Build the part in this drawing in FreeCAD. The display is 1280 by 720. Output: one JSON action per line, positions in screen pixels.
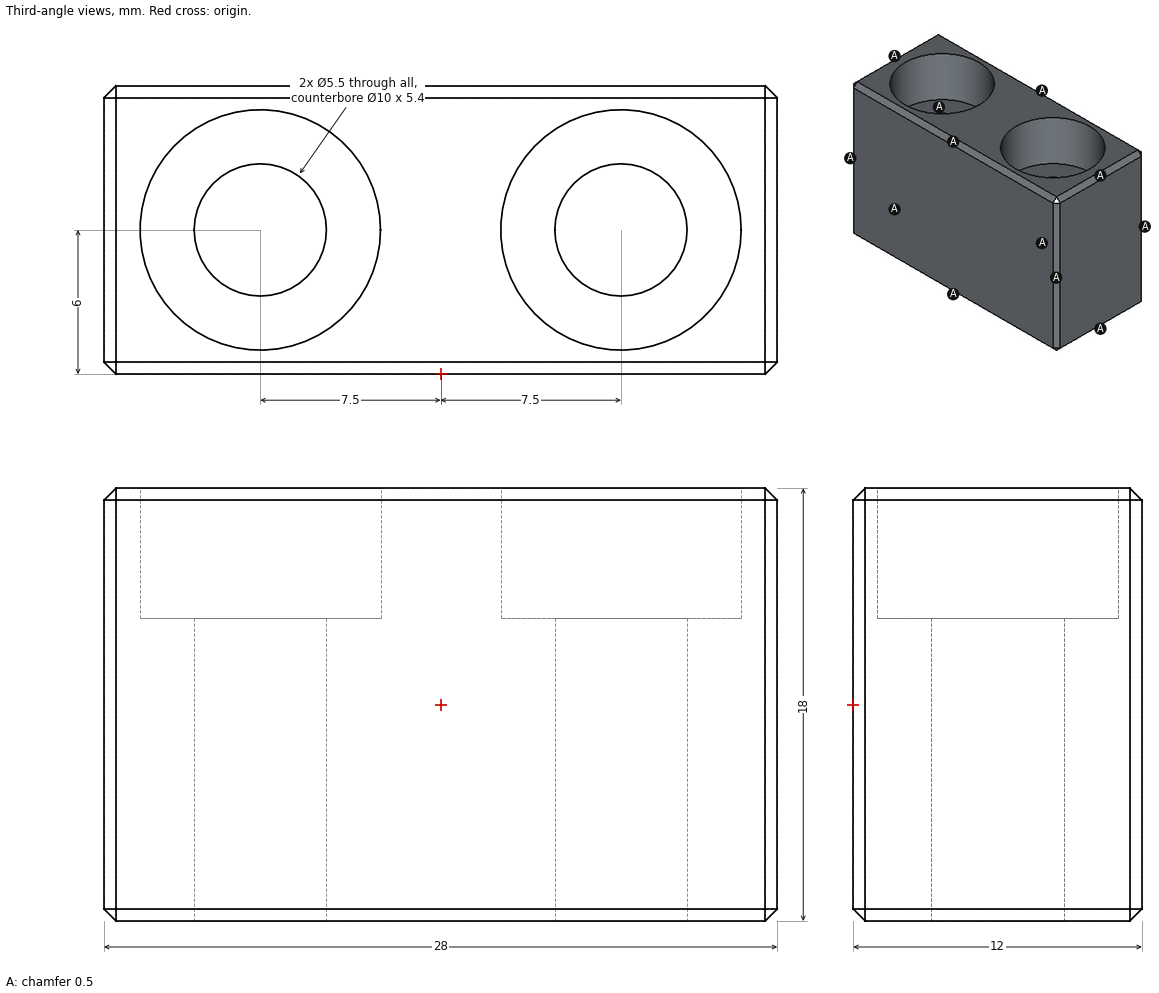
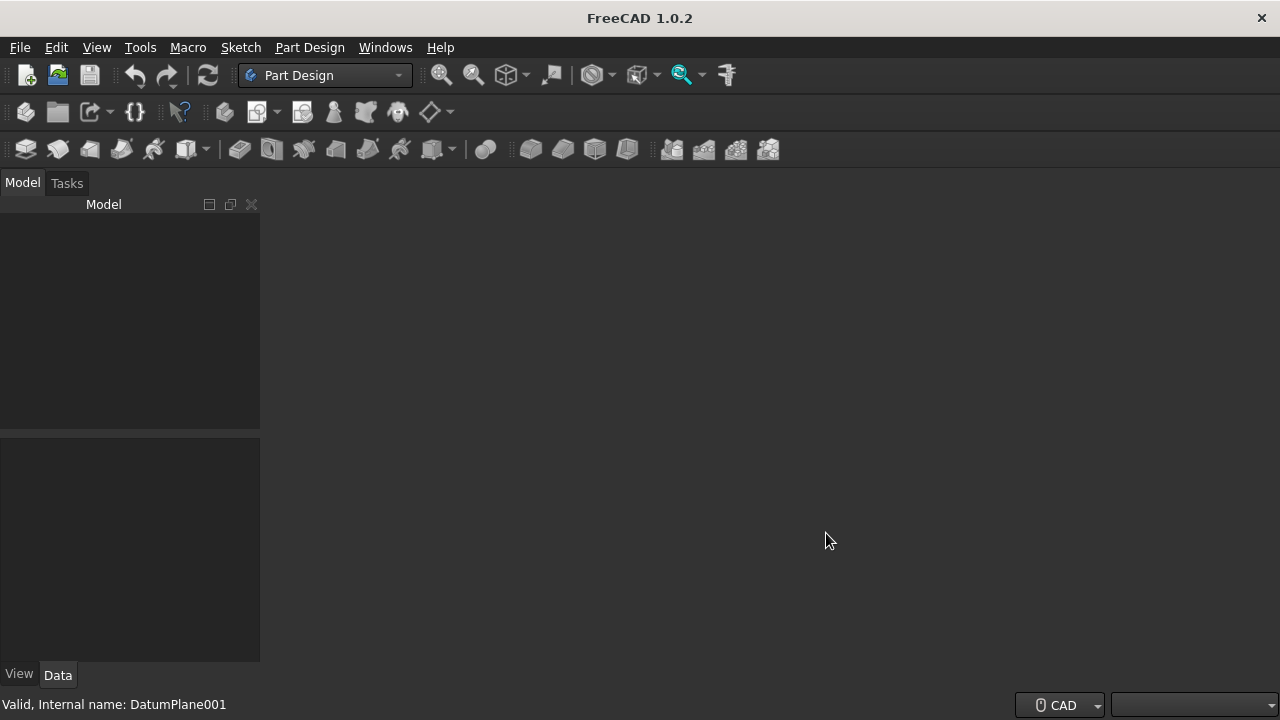
{"action": "left_click", "coordinate": [26, 76]}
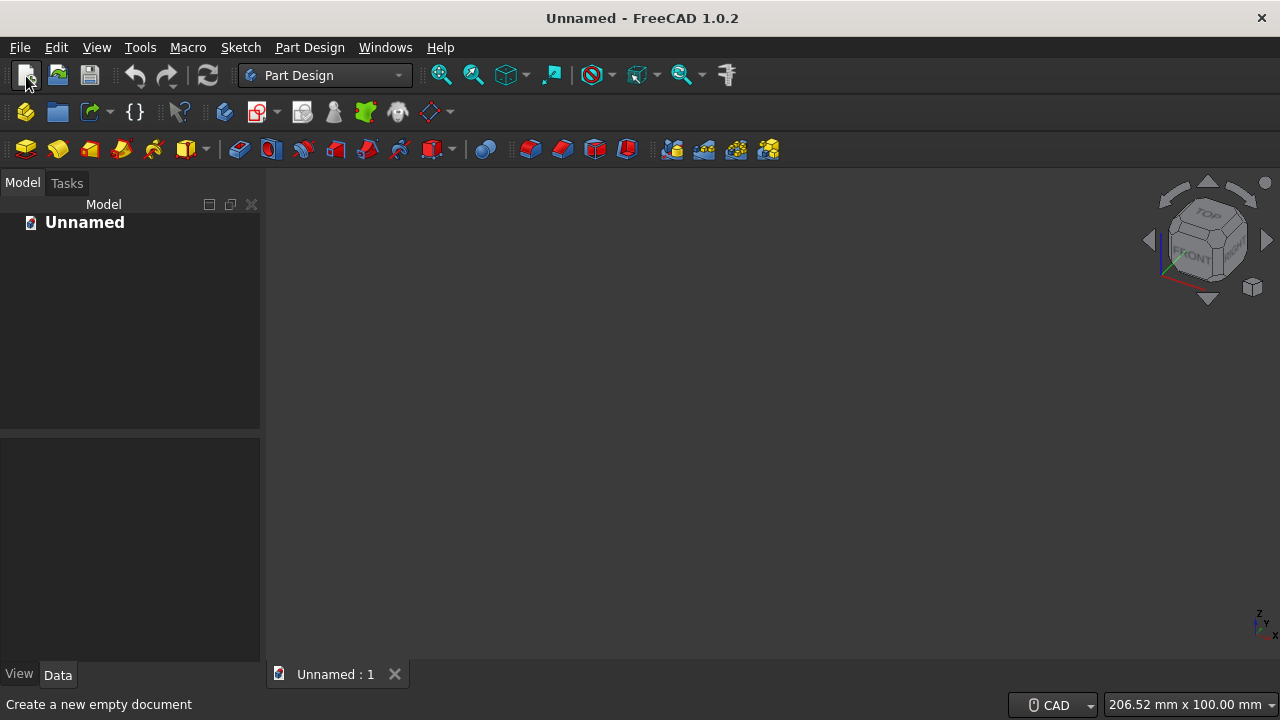
{"action": "left_click", "coordinate": [258, 112]}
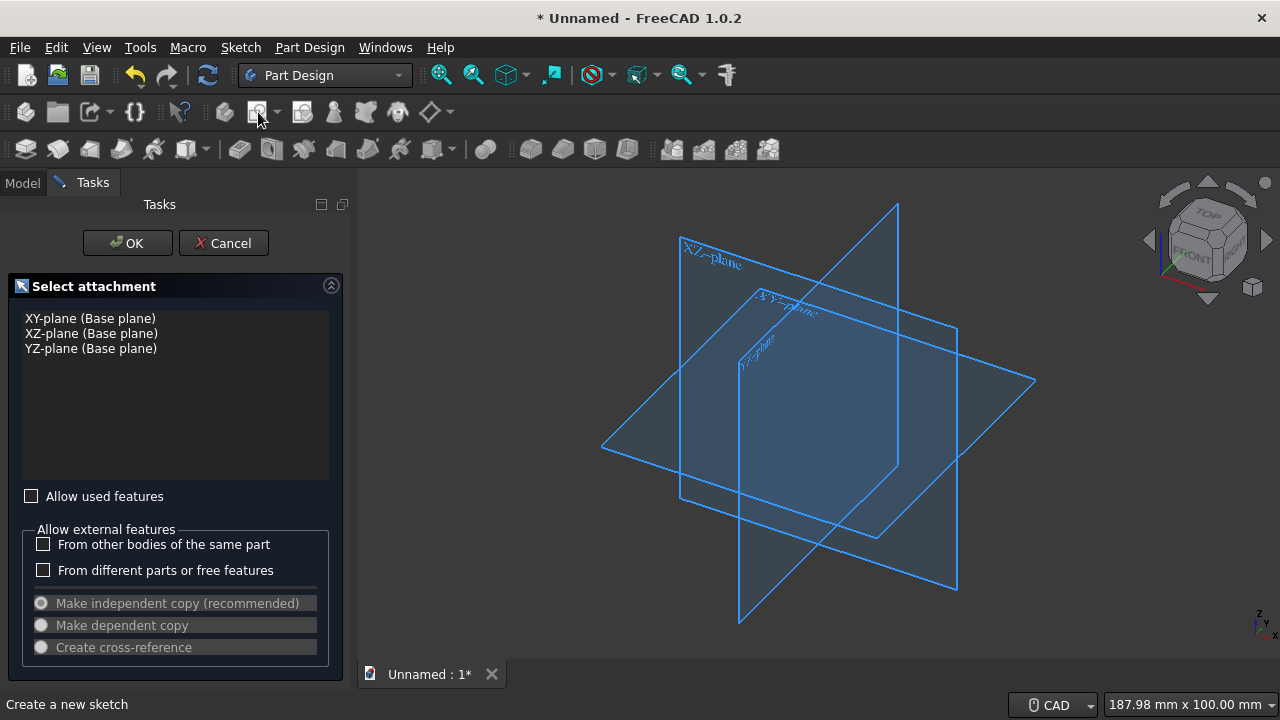
{"action": "left_click", "coordinate": [82, 334]}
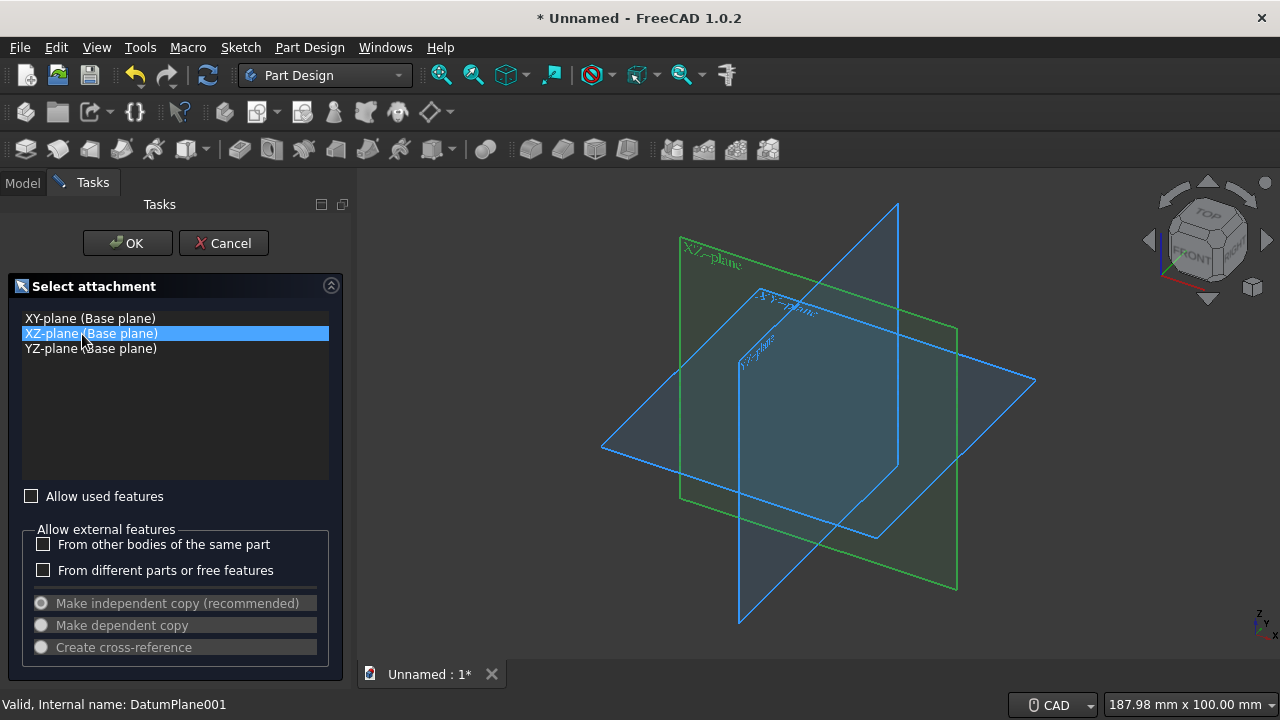
{"action": "left_click", "coordinate": [128, 243]}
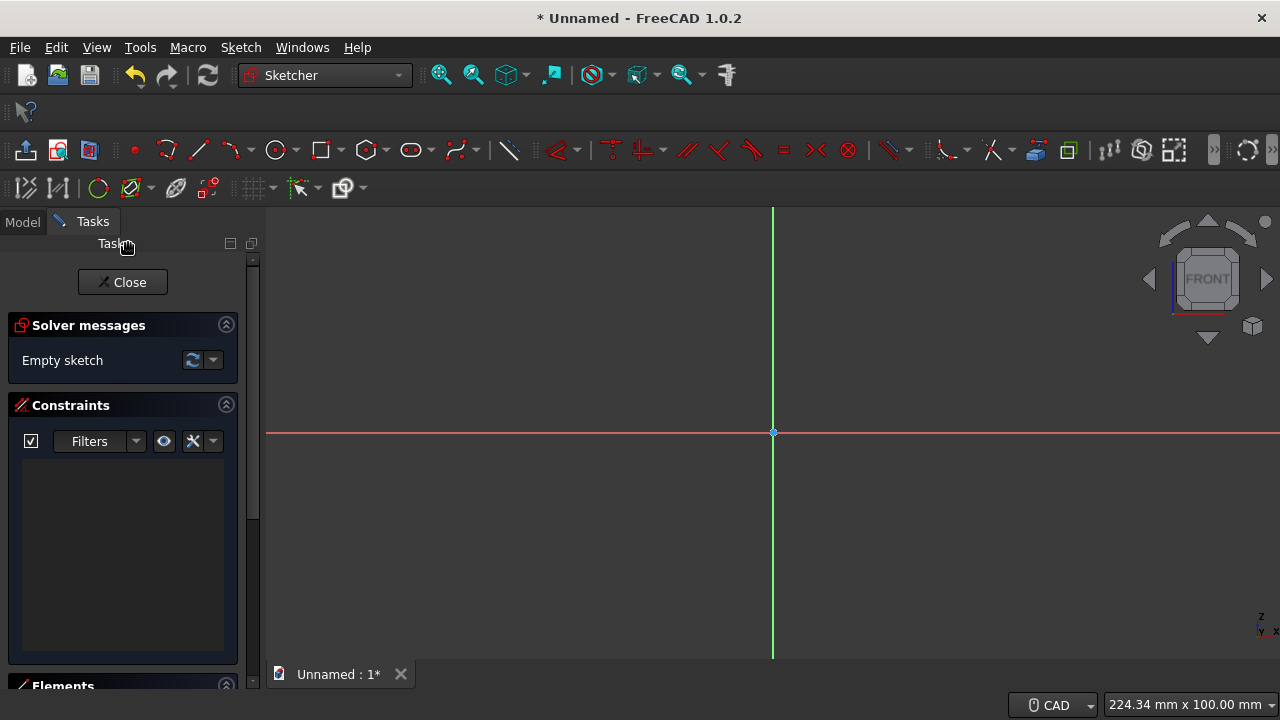
{"action": "scroll", "coordinate": [803, 433], "scroll_direction": "up", "scroll_amount": 6}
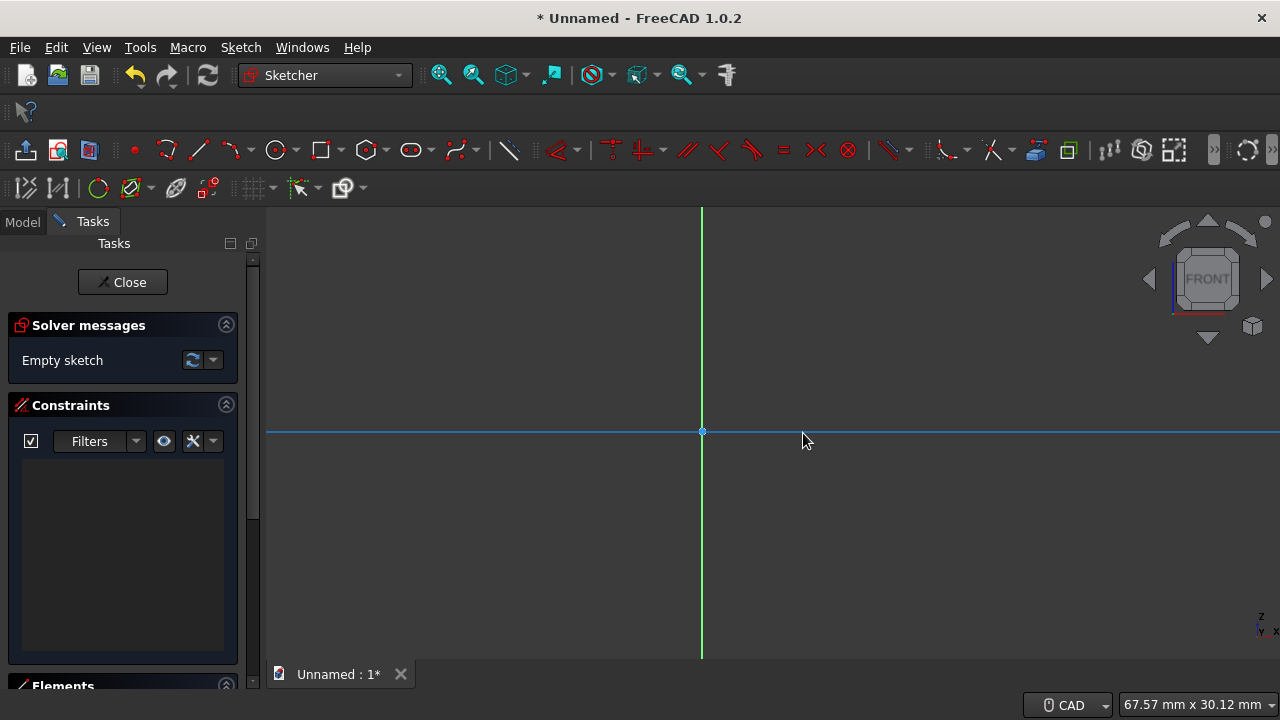
{"action": "key", "text": "g v"}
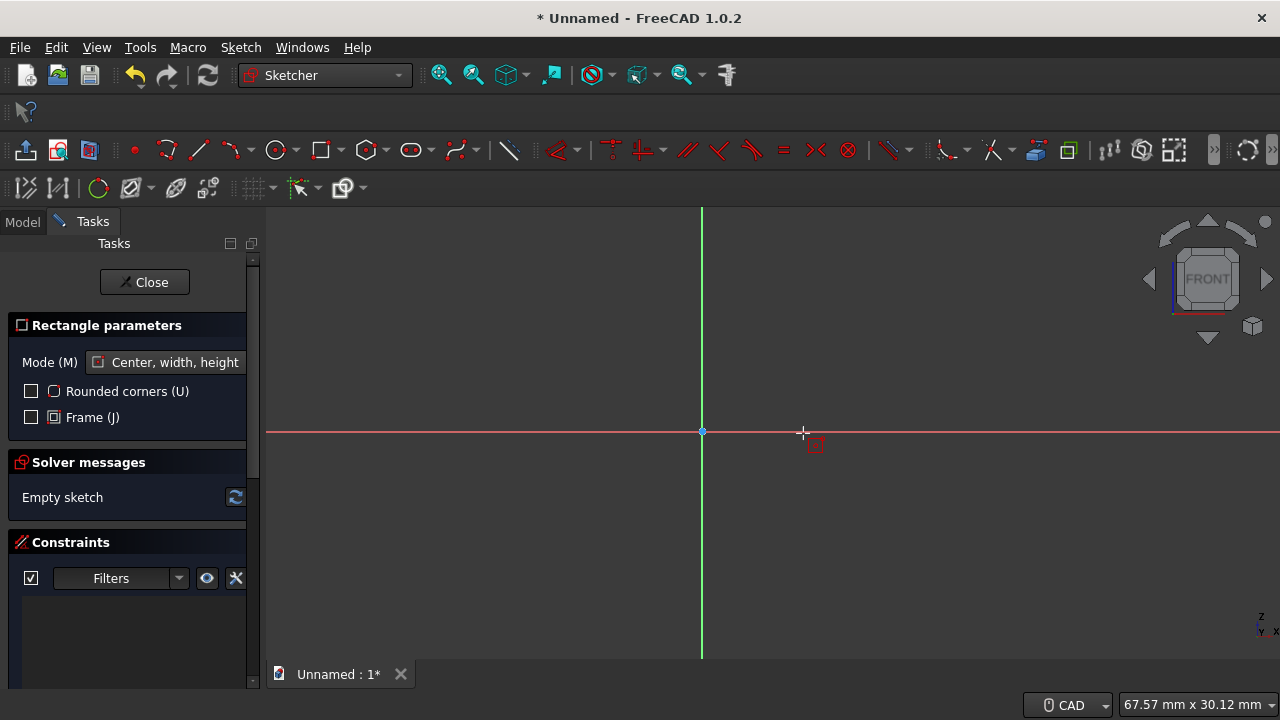
{"action": "left_click", "coordinate": [702, 432]}
{"action": "mouse_move", "coordinate": [912, 297]}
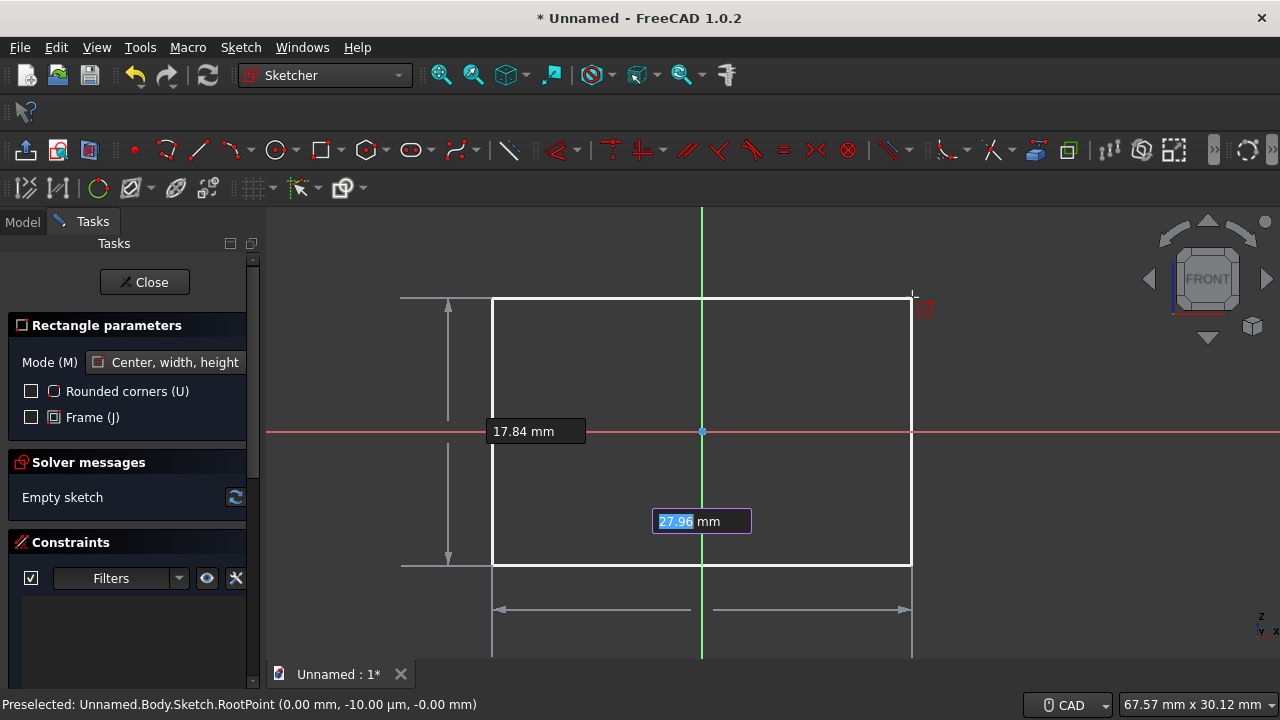
{"action": "type", "text": "28"}
{"action": "key", "text": "Tab"}
{"action": "type", "text": "18"}
{"action": "key", "text": "Return"}
{"action": "key", "text": "Escape"}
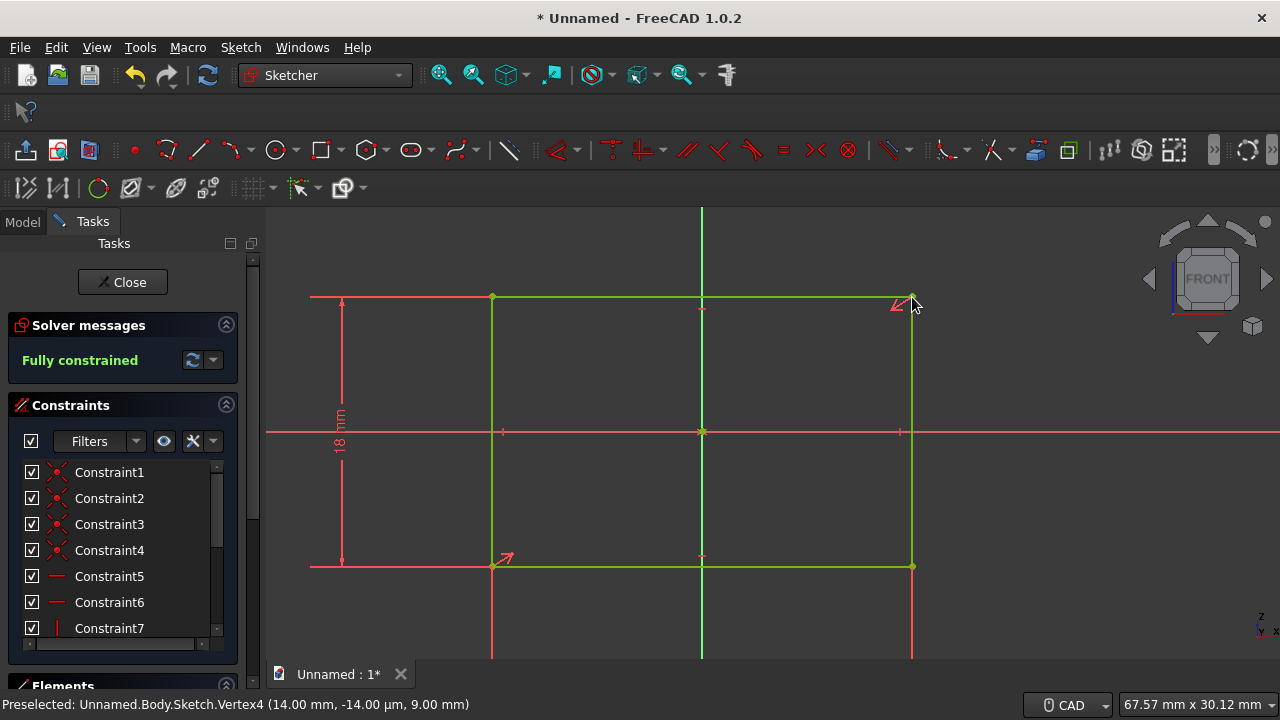
{"action": "left_click", "coordinate": [123, 282]}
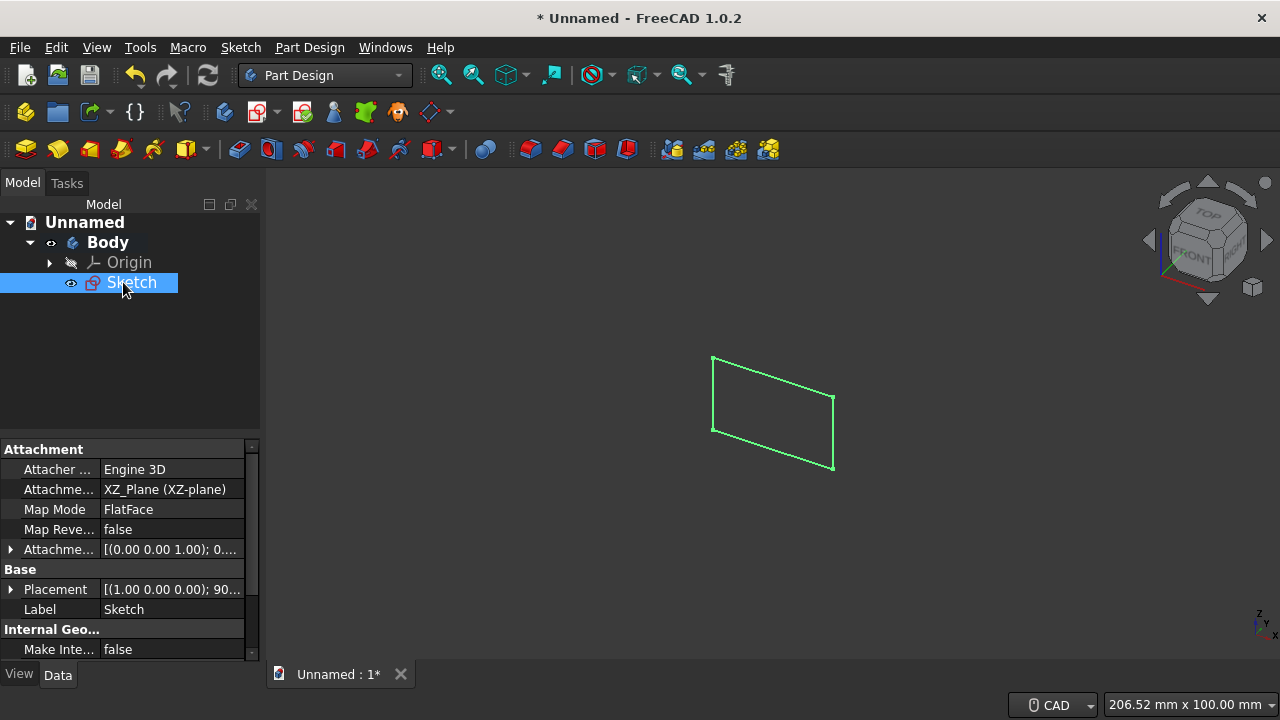
{"action": "left_click", "coordinate": [26, 150]}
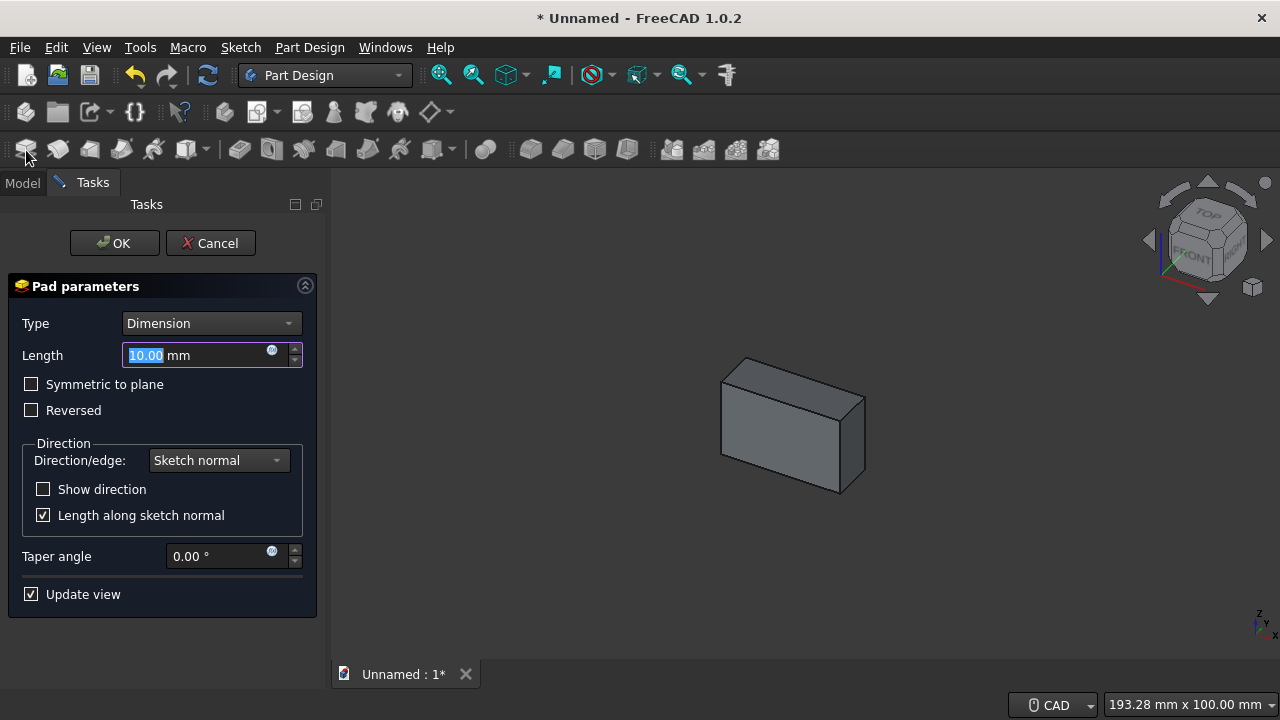
{"action": "type", "text": "12"}
{"action": "key", "text": "Tab"}